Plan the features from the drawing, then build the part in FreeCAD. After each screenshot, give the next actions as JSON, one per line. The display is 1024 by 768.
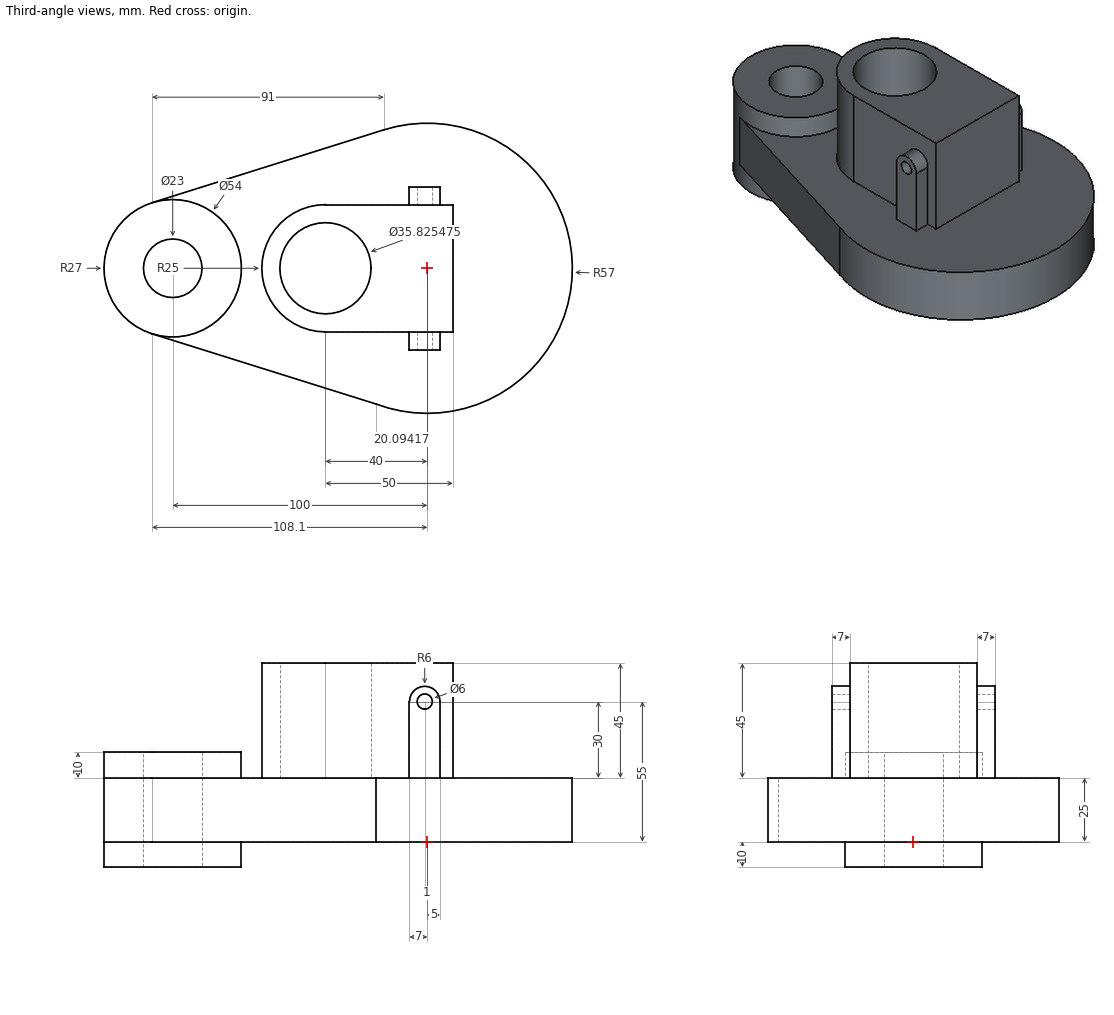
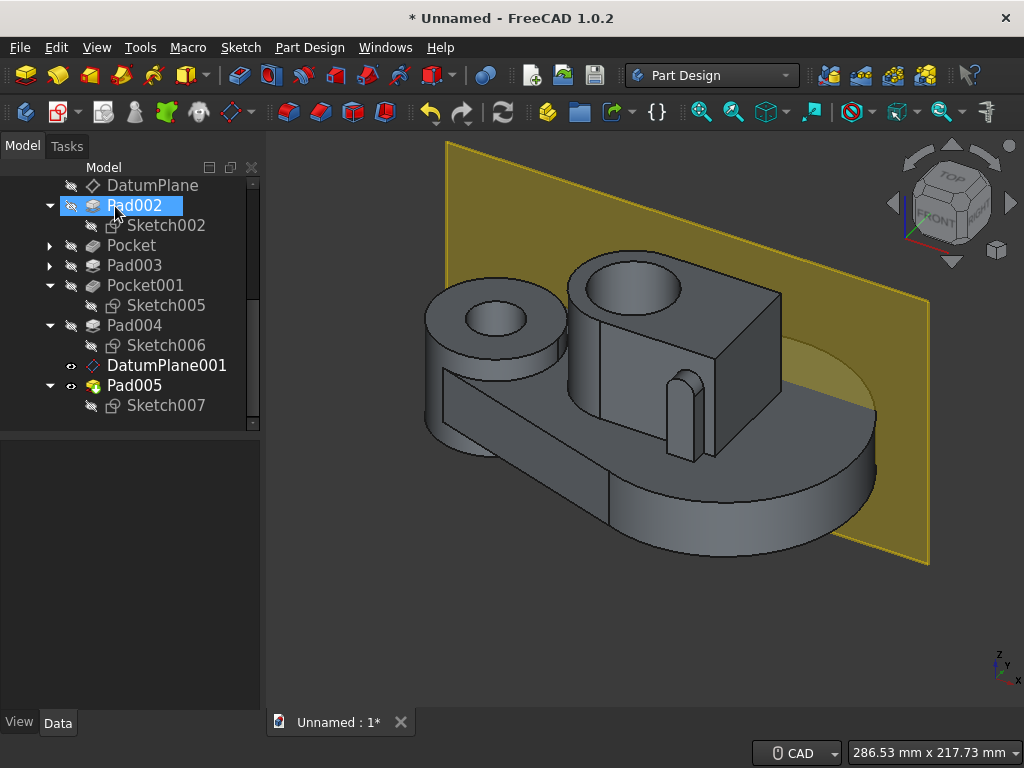
{"action": "left_click", "coordinate": [116, 366]}
{"action": "key", "text": "space"}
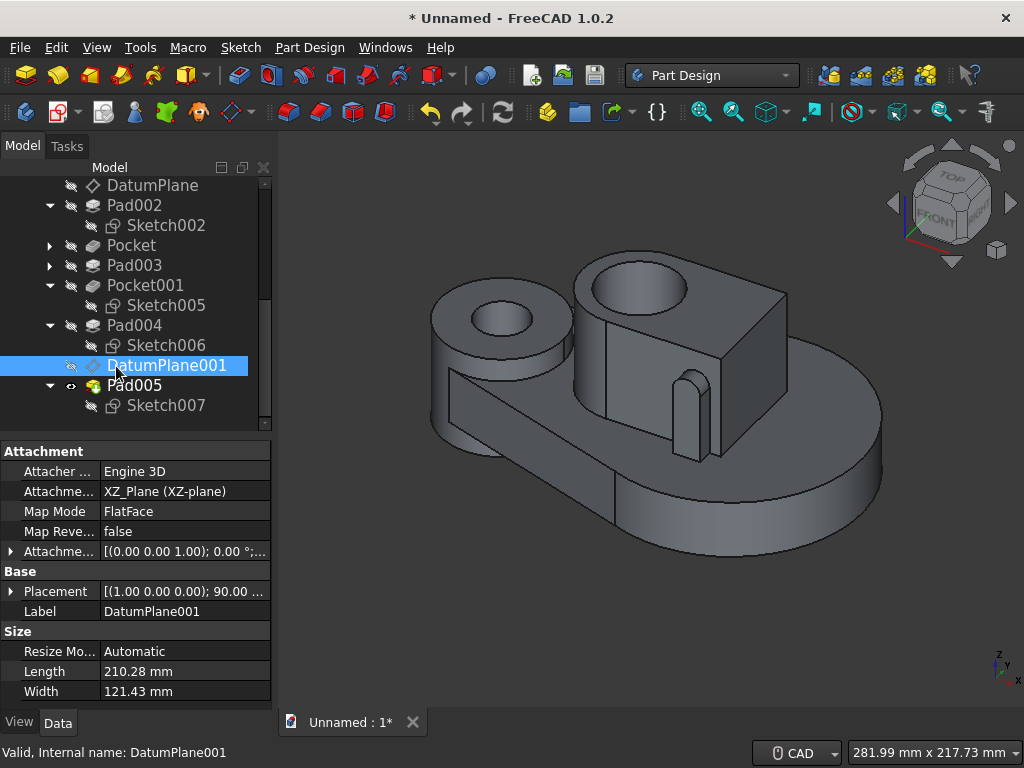
{"action": "left_click", "coordinate": [687, 395]}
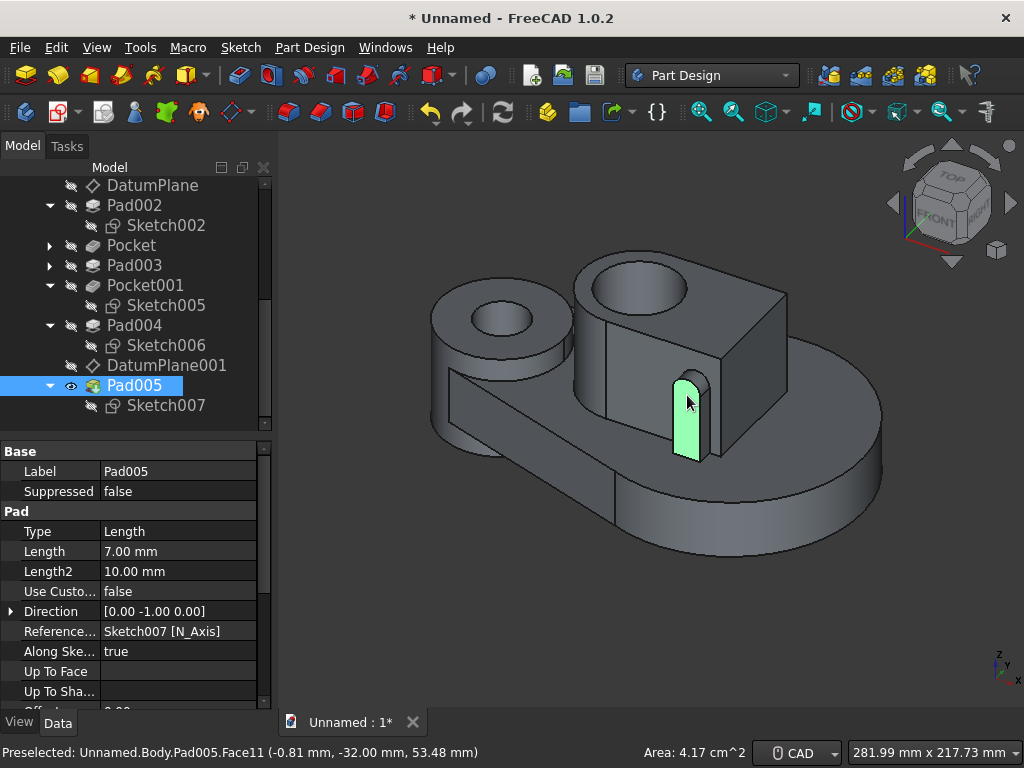
{"action": "left_click", "coordinate": [58, 112]}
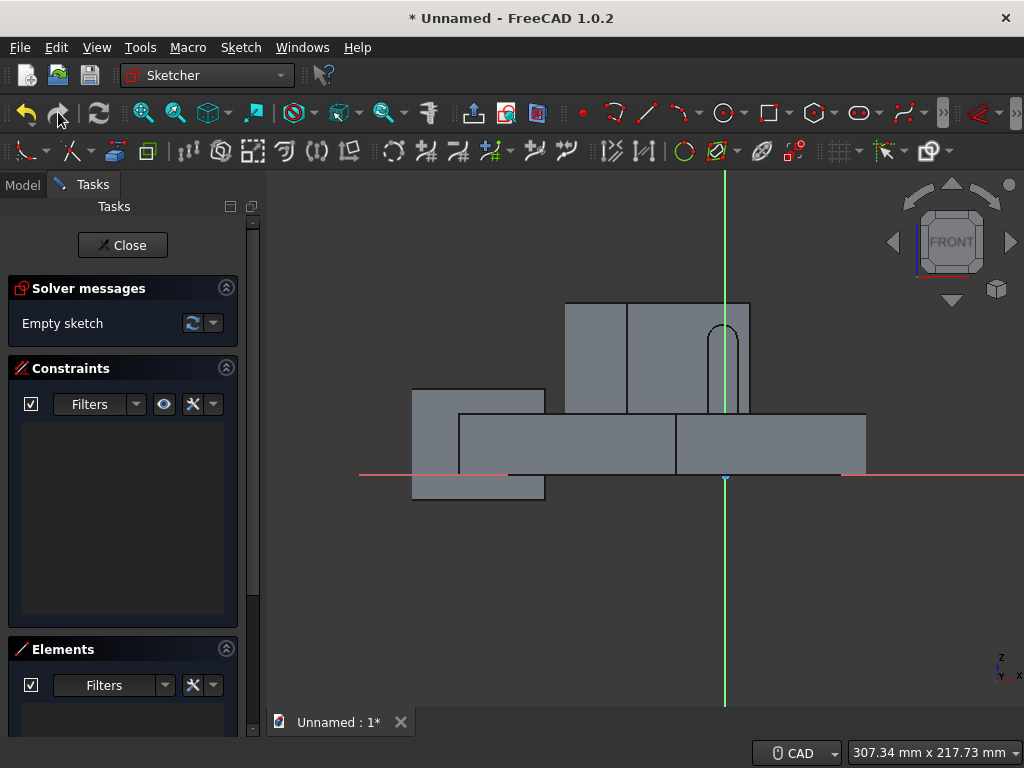
{"action": "key", "text": "q s"}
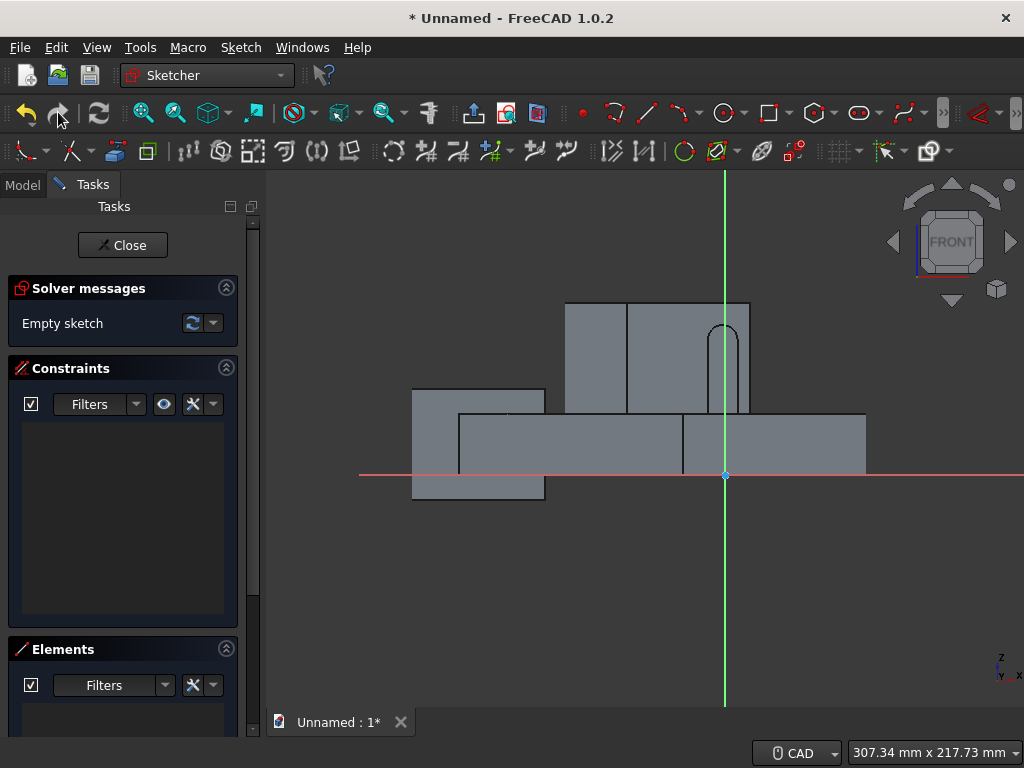
{"action": "scroll", "coordinate": [730, 335], "scroll_direction": "up", "scroll_amount": 15}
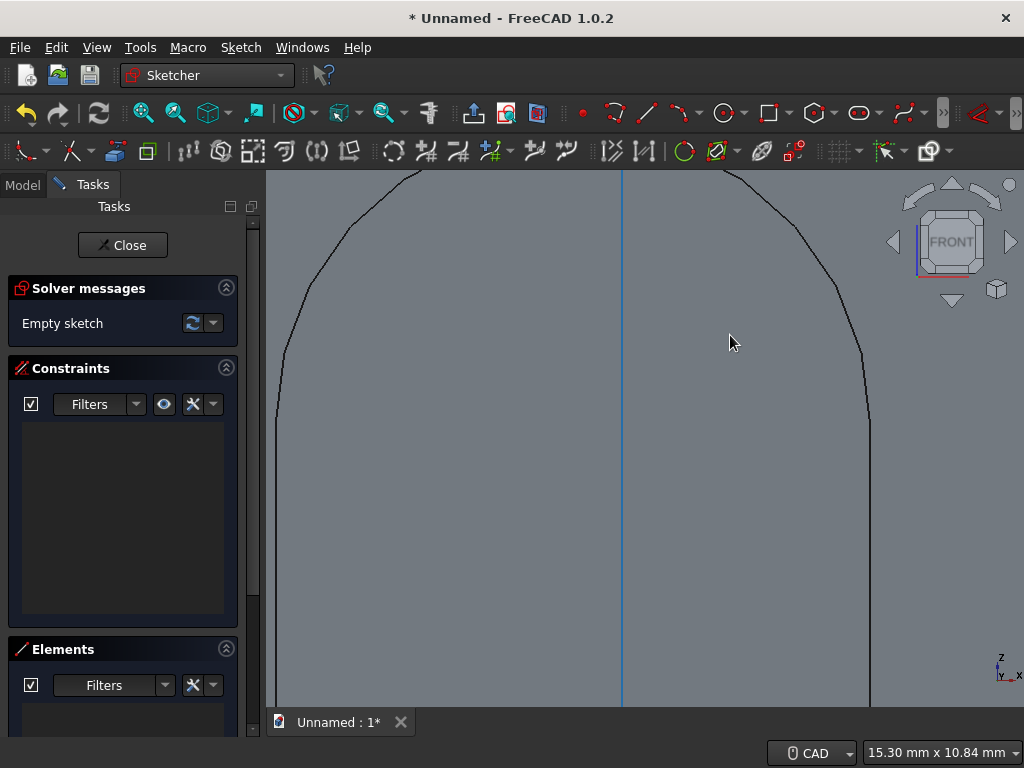
{"action": "key", "text": "g c"}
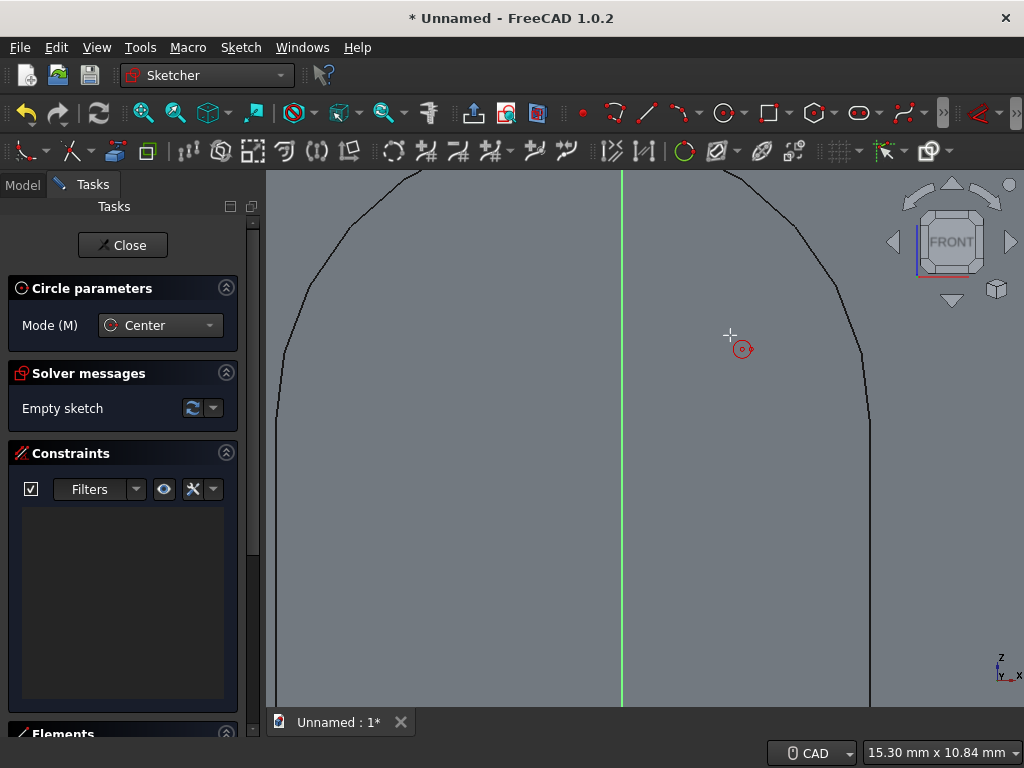
{"action": "left_click", "coordinate": [573, 424]}
{"action": "left_click", "coordinate": [678, 319]}
{"action": "key", "text": "Escape"}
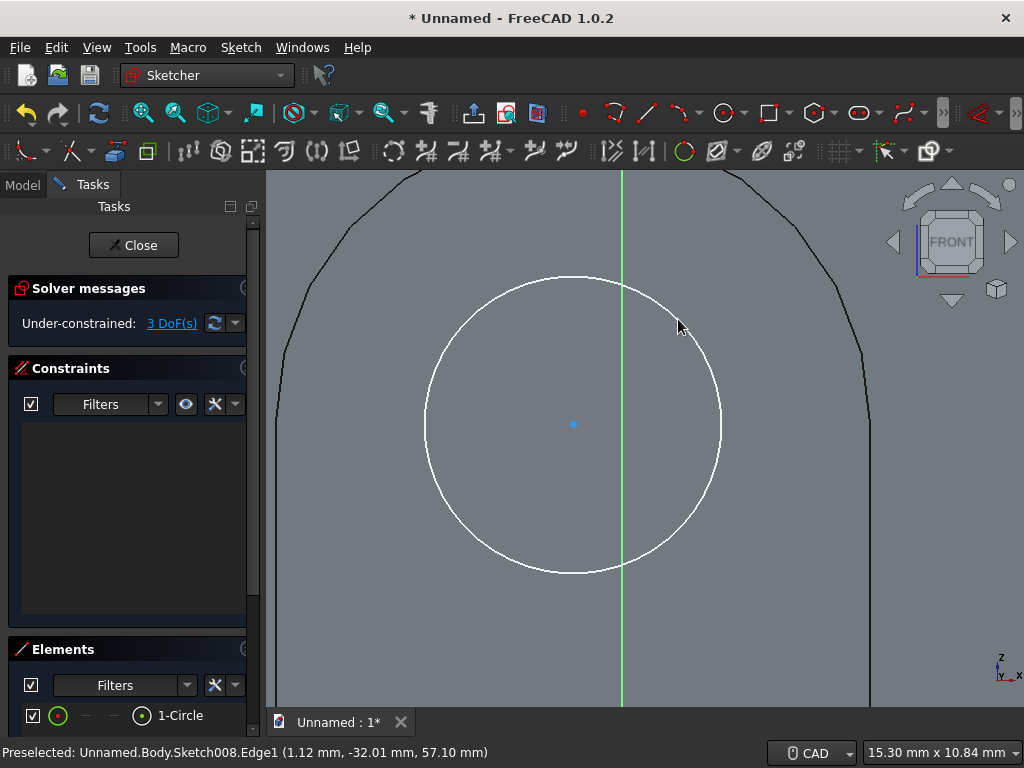
{"action": "key", "text": "d"}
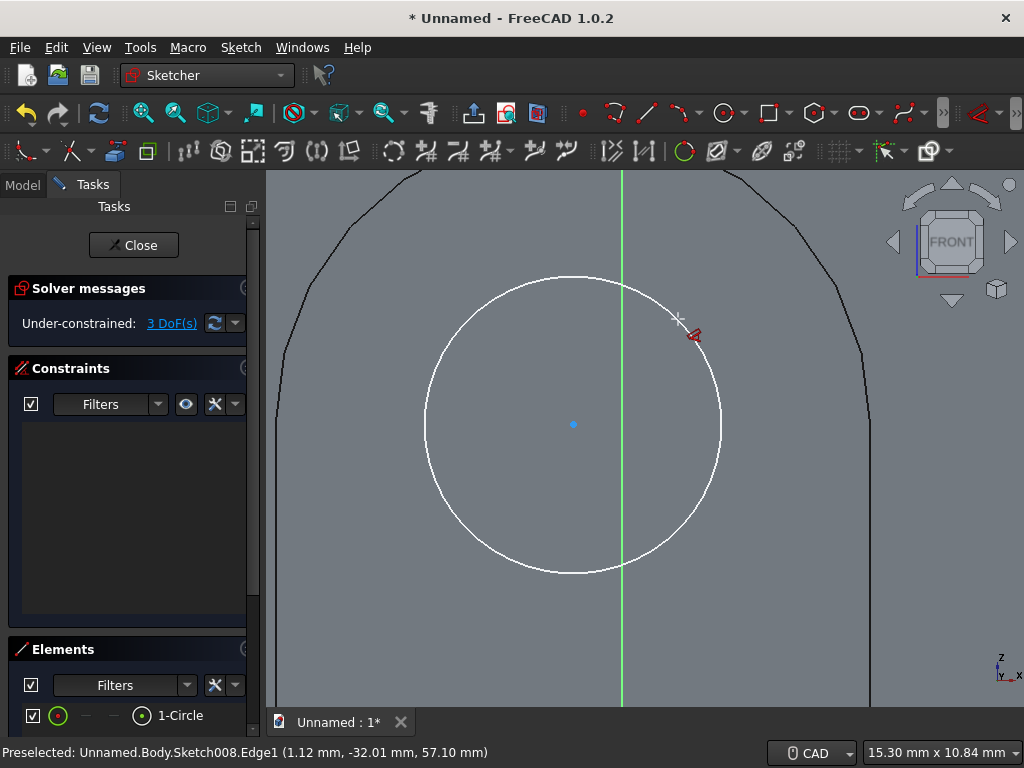
{"action": "left_click", "coordinate": [678, 320]}
{"action": "left_click", "coordinate": [701, 297]}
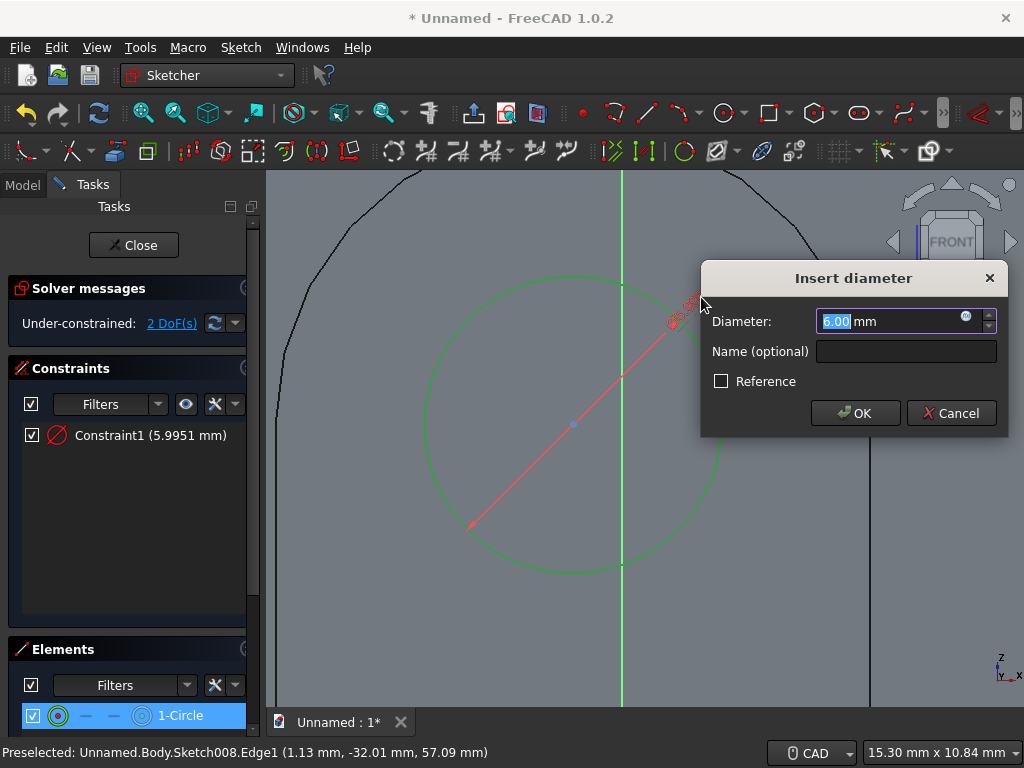
{"action": "type", "text": "6"}
{"action": "key", "text": "Return"}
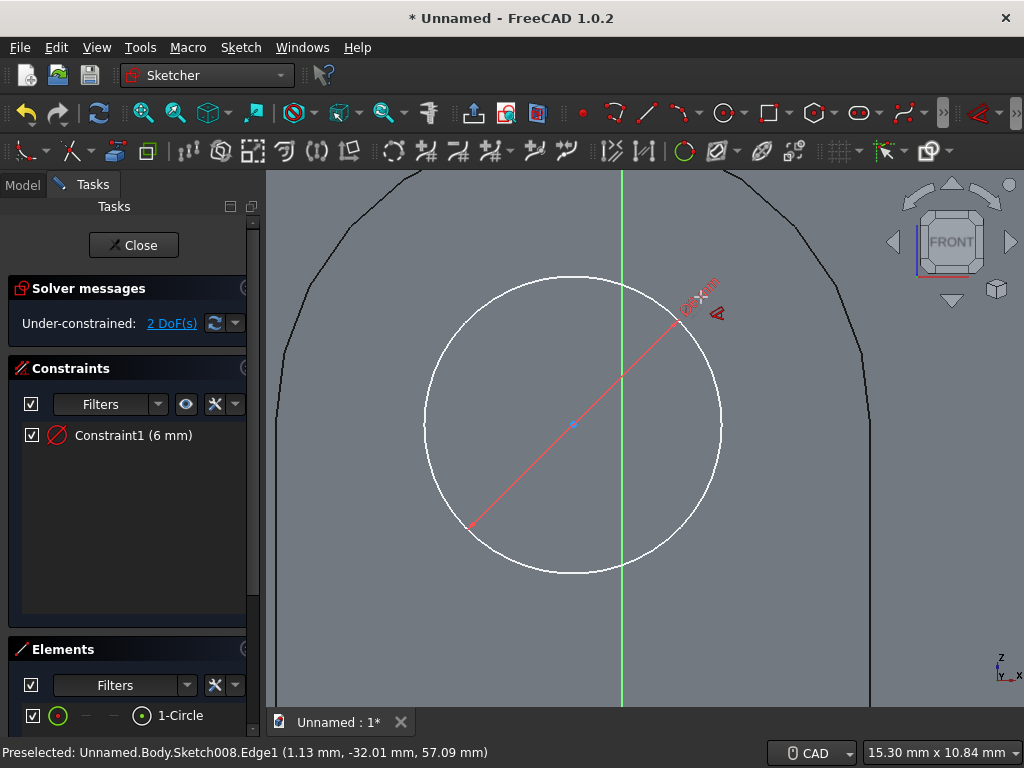
{"action": "left_click", "coordinate": [573, 425]}
{"action": "left_click", "coordinate": [598, 391]}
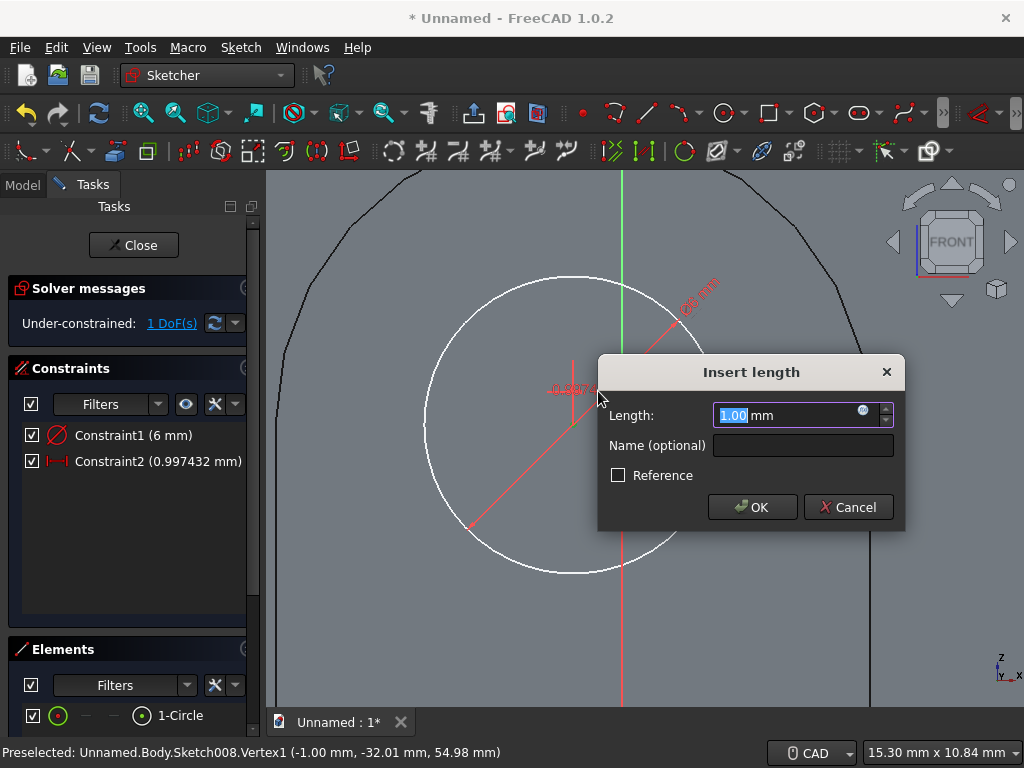
{"action": "type", "text": "1"}
{"action": "key", "text": "Return"}